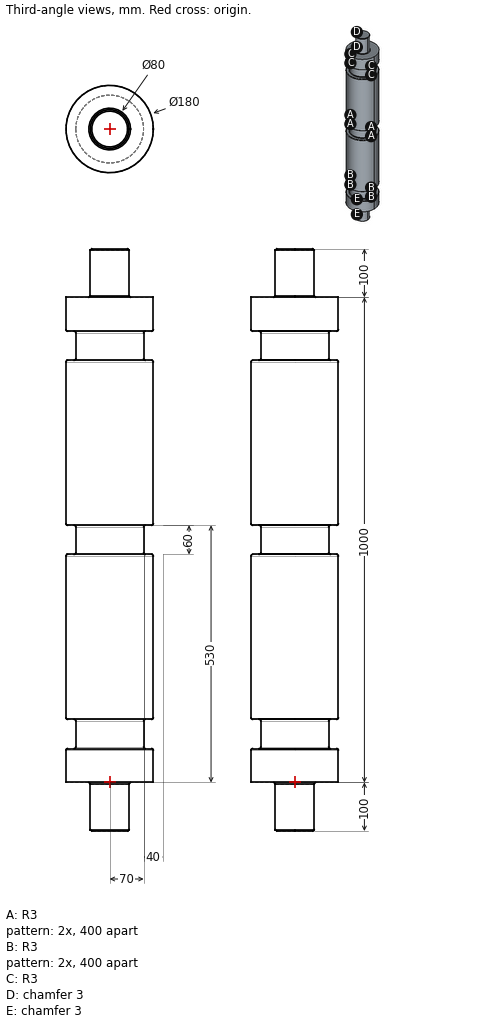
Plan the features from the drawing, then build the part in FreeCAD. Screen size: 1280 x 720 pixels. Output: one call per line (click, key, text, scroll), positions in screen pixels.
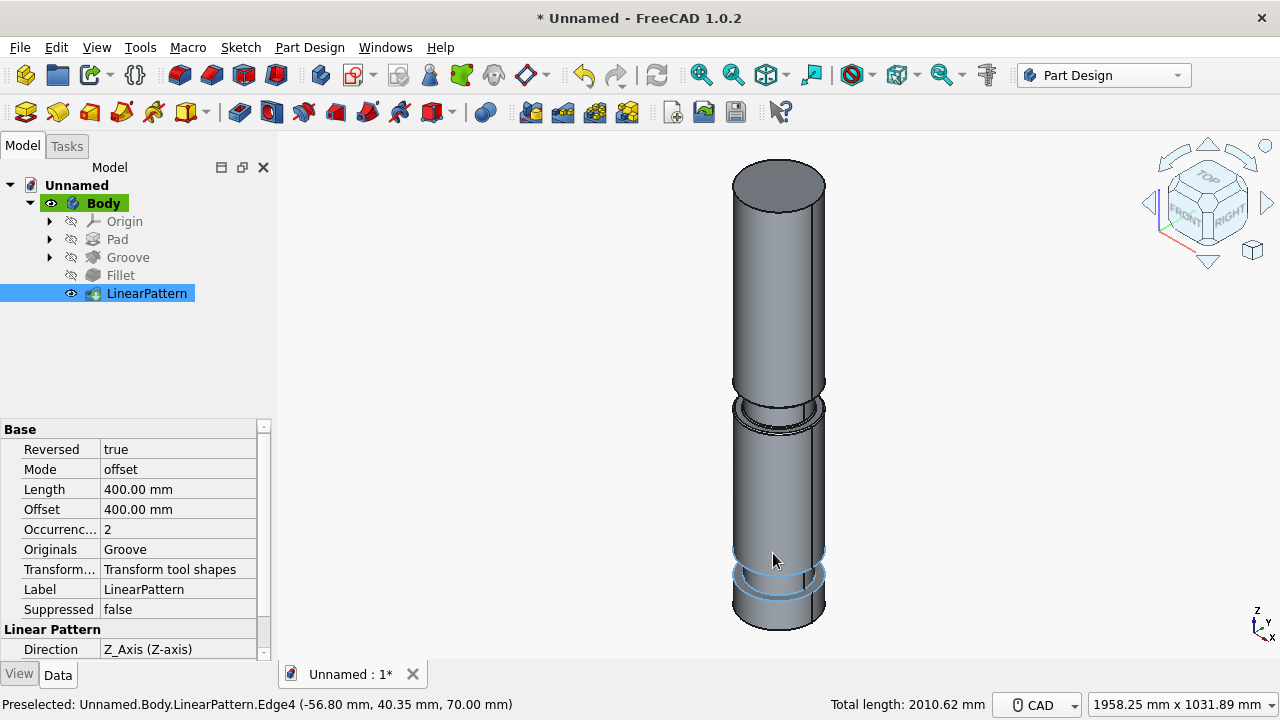
click(180, 76)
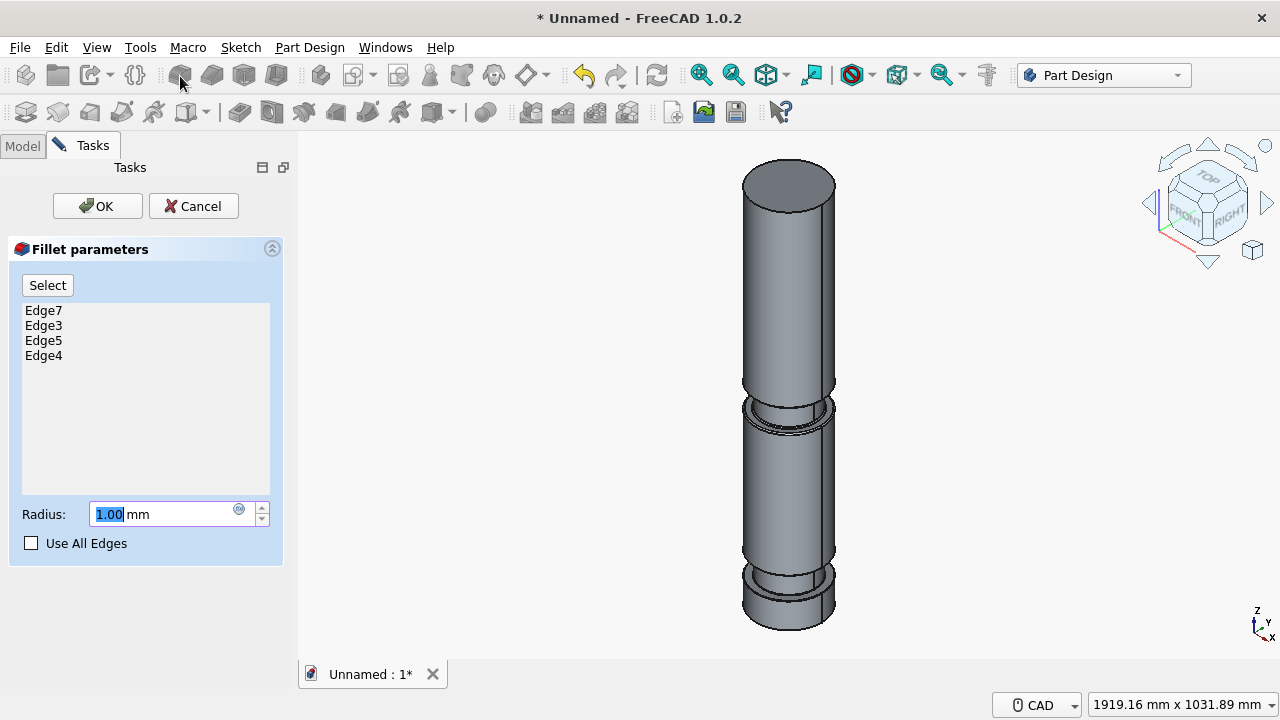
text(3)
key(Tab)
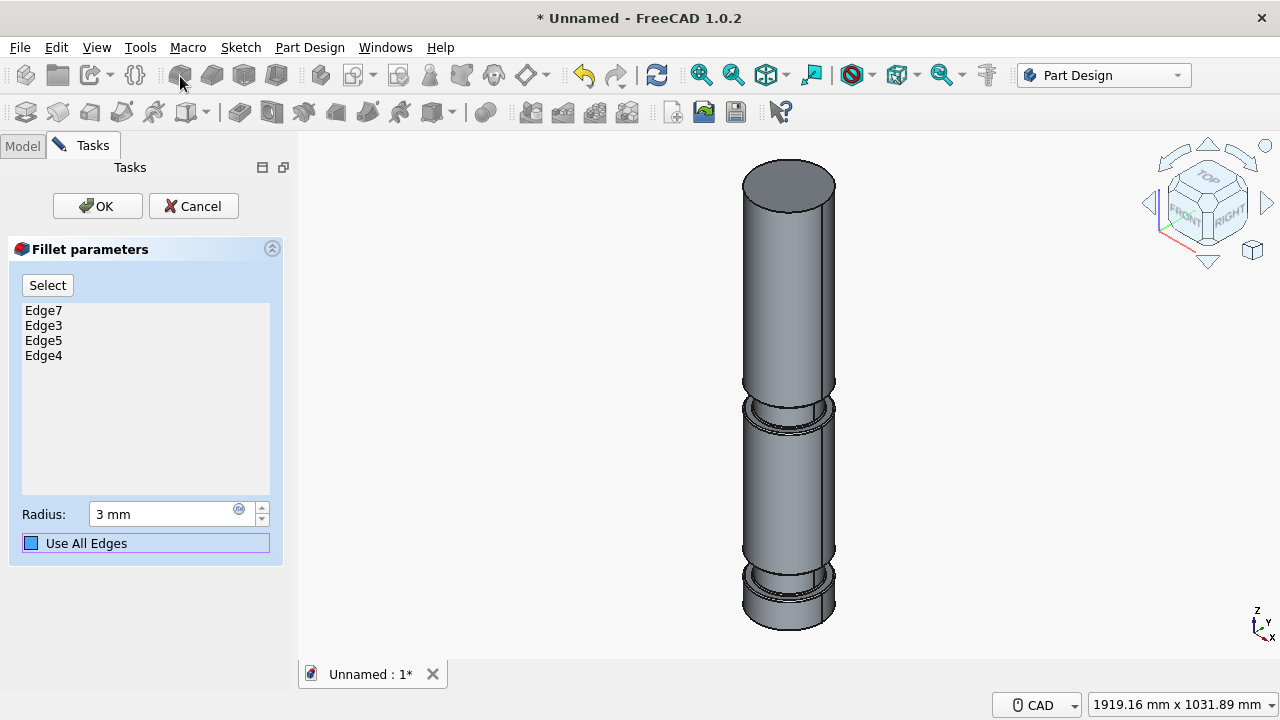
click(98, 206)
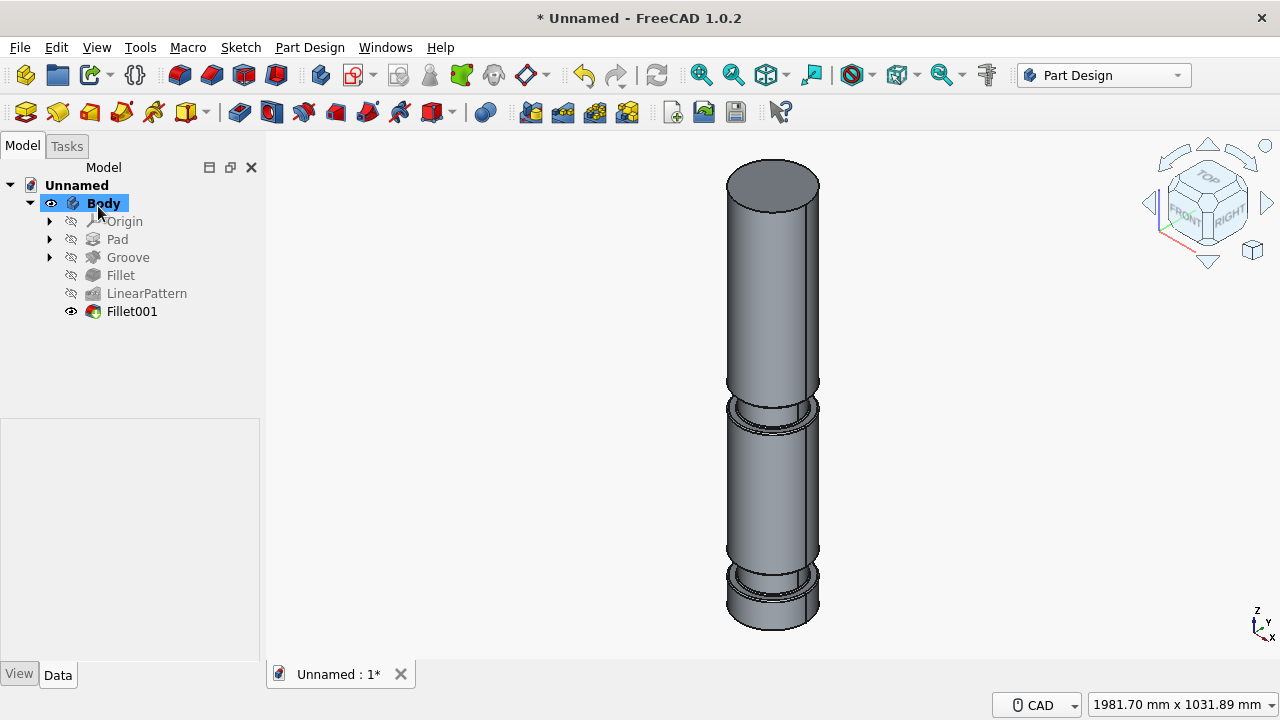
click(116, 257)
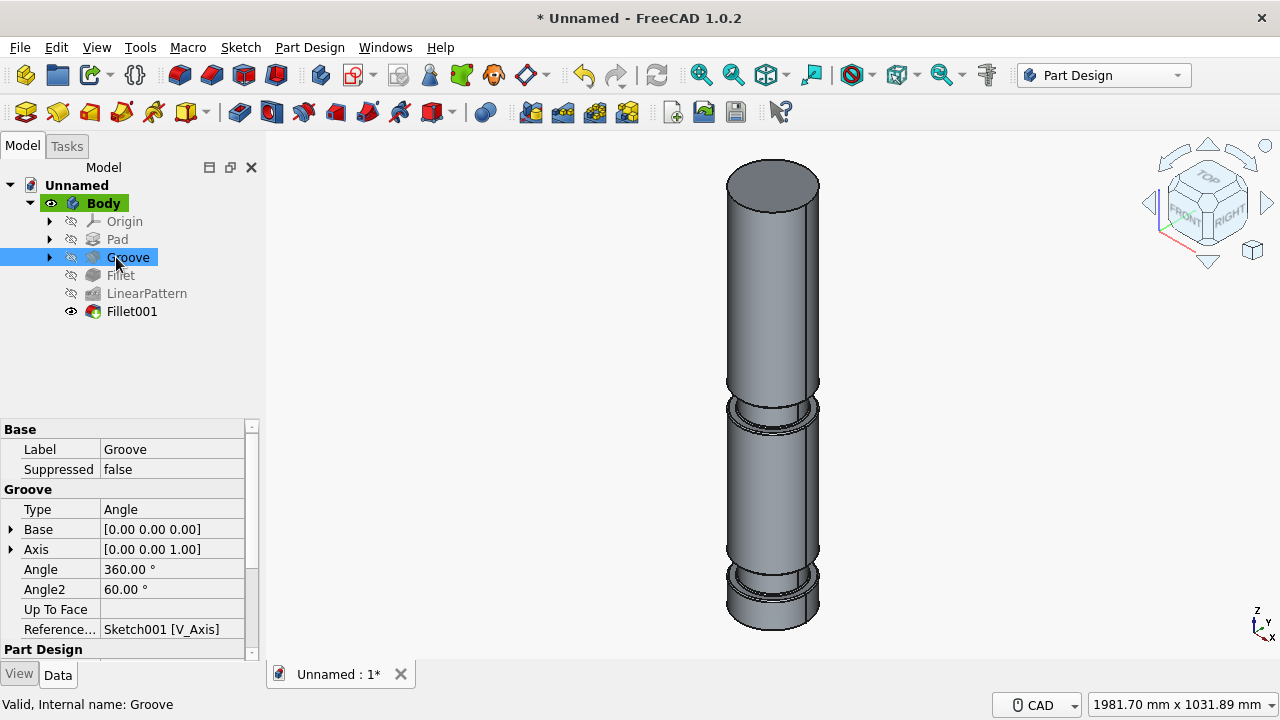
click(564, 112)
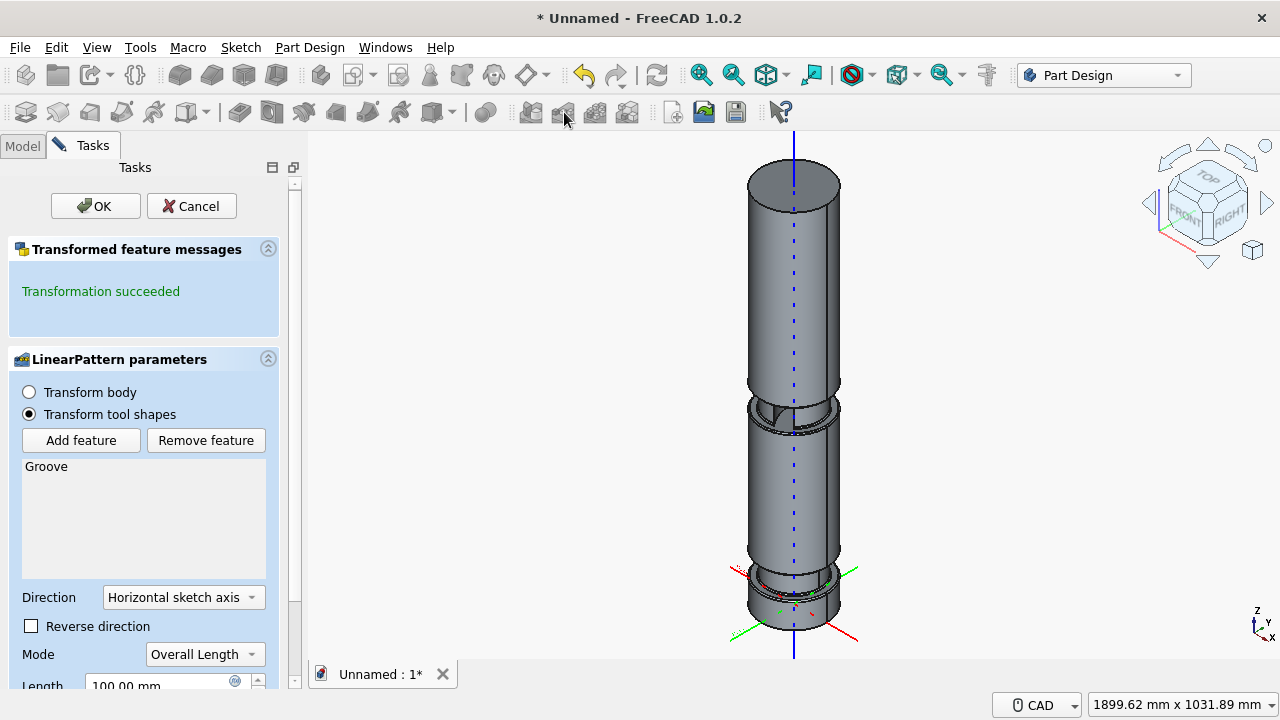
click(184, 598)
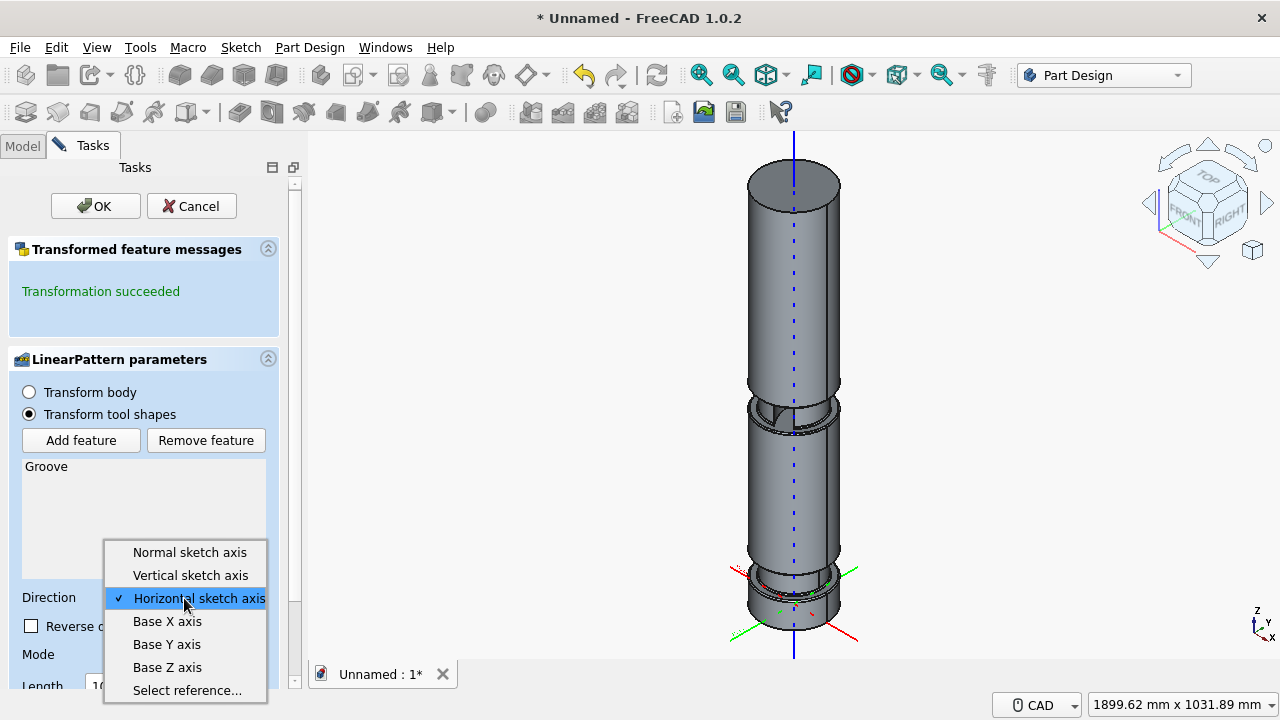
click(184, 668)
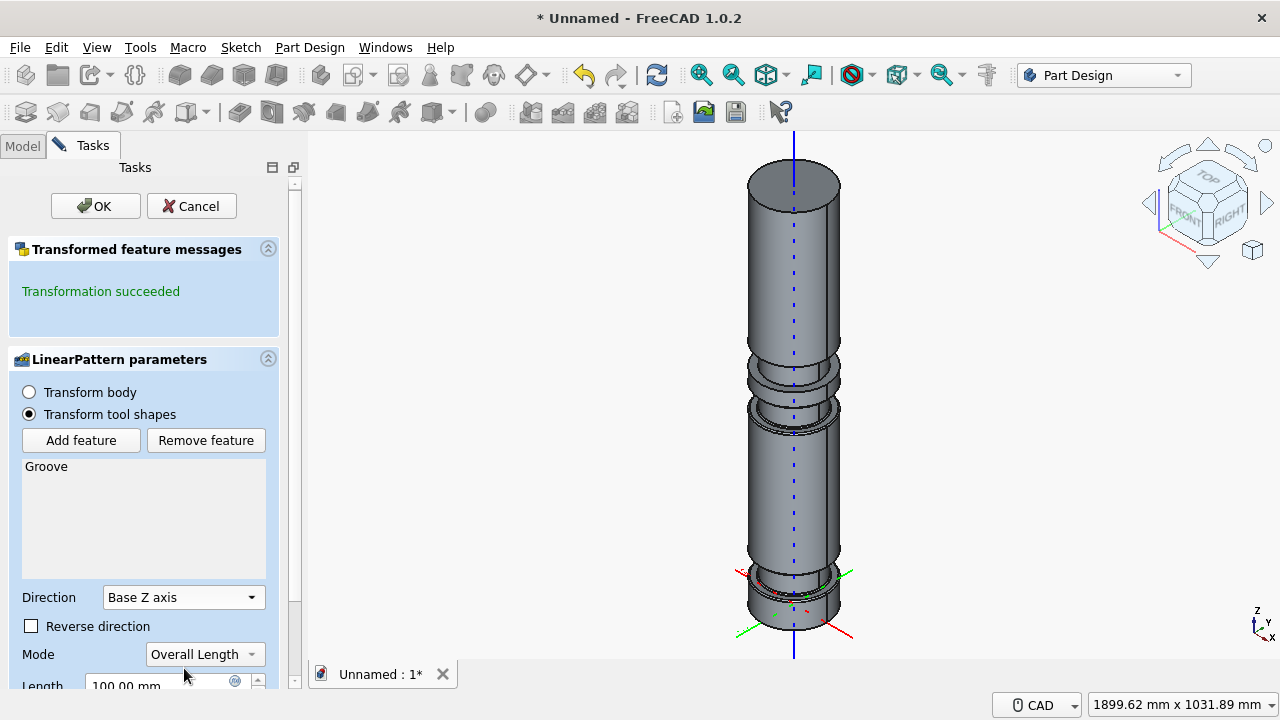
click(206, 654)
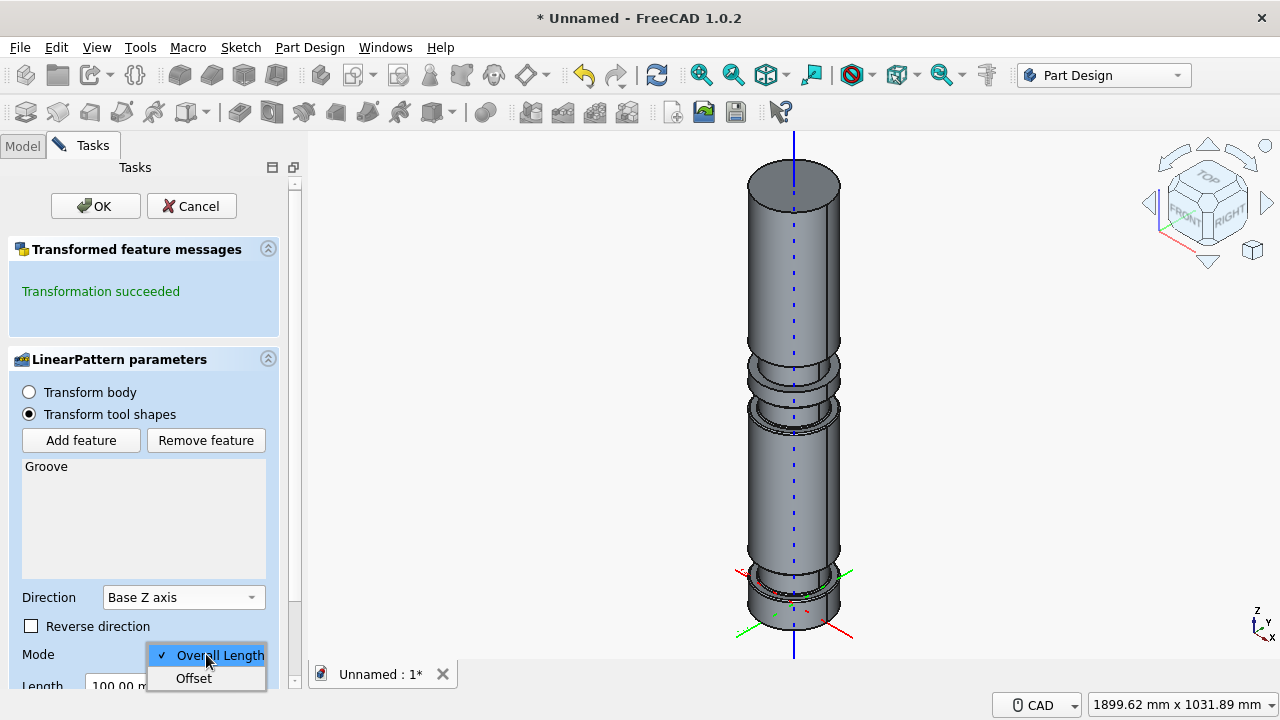
click(206, 678)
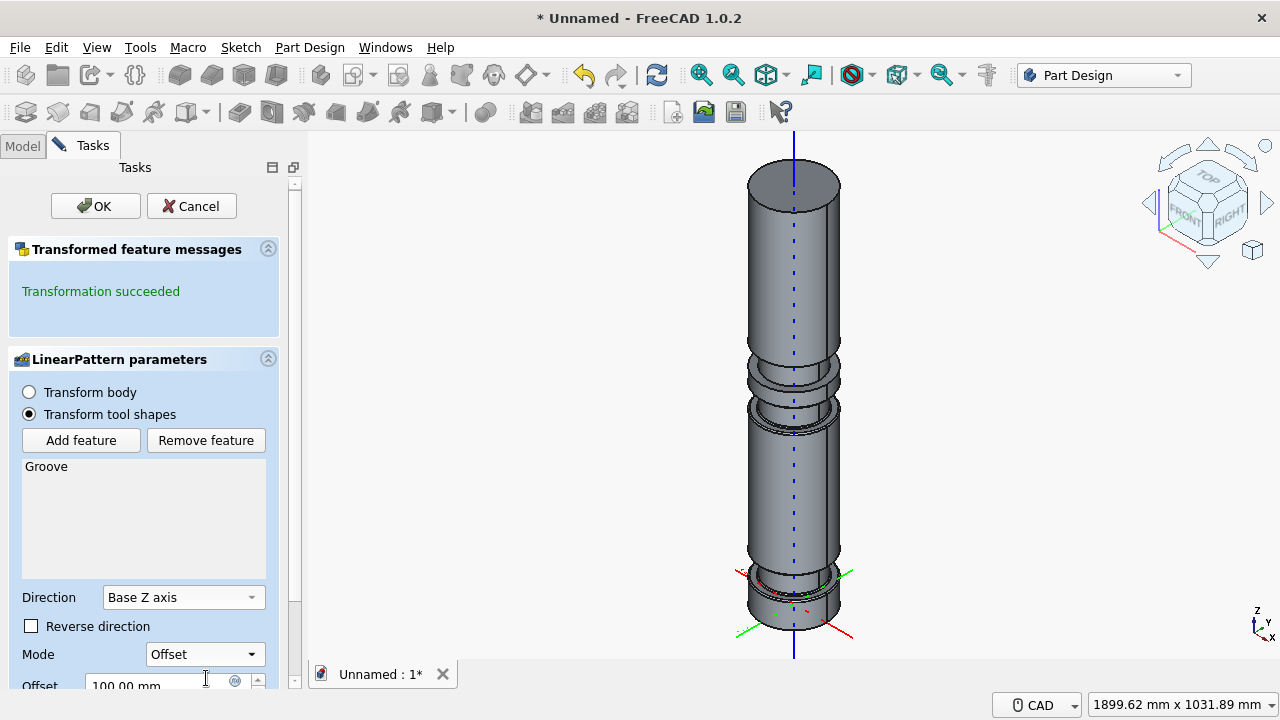
scroll(295, 432, down, 2)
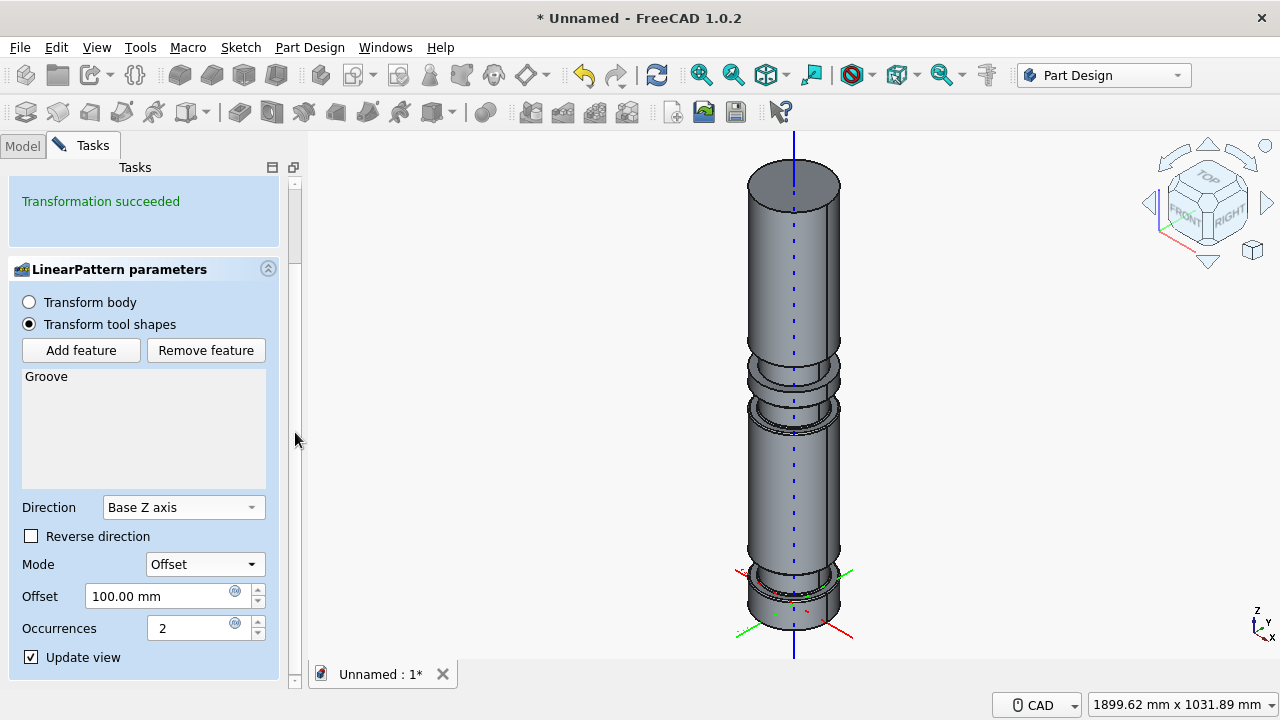
triple_click(168, 596)